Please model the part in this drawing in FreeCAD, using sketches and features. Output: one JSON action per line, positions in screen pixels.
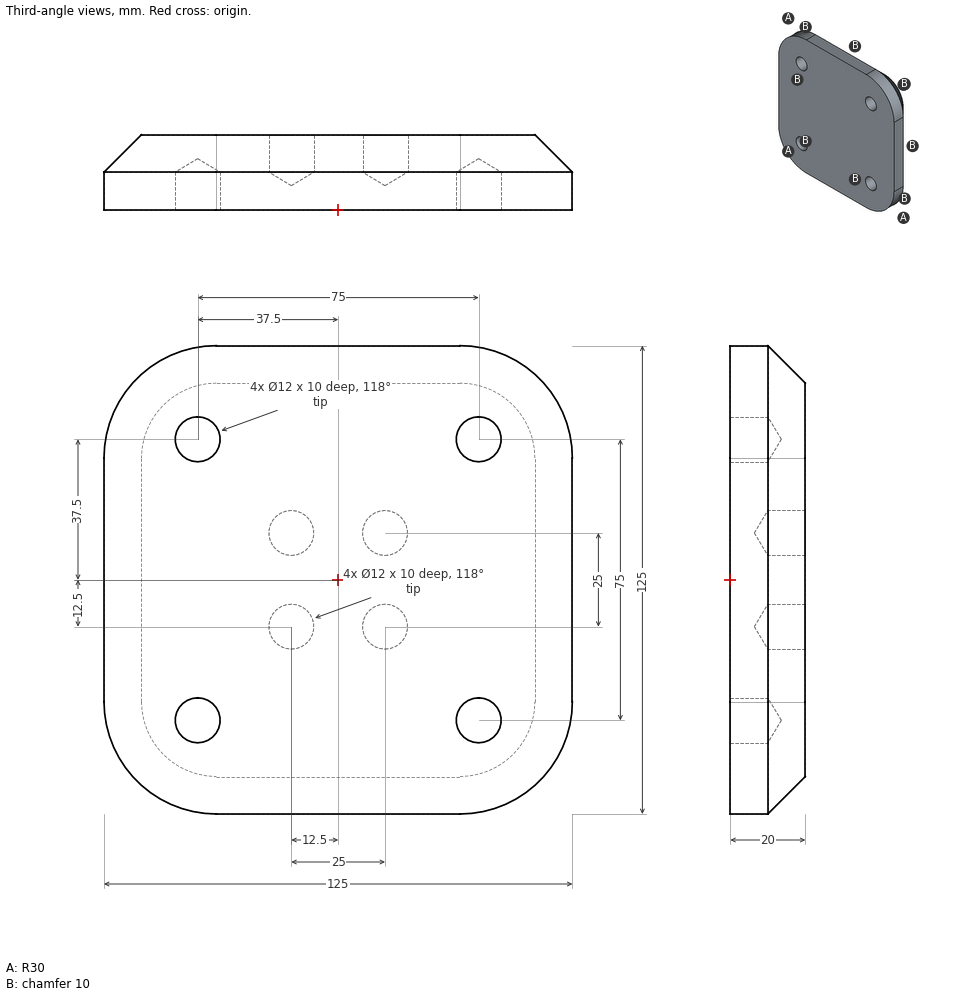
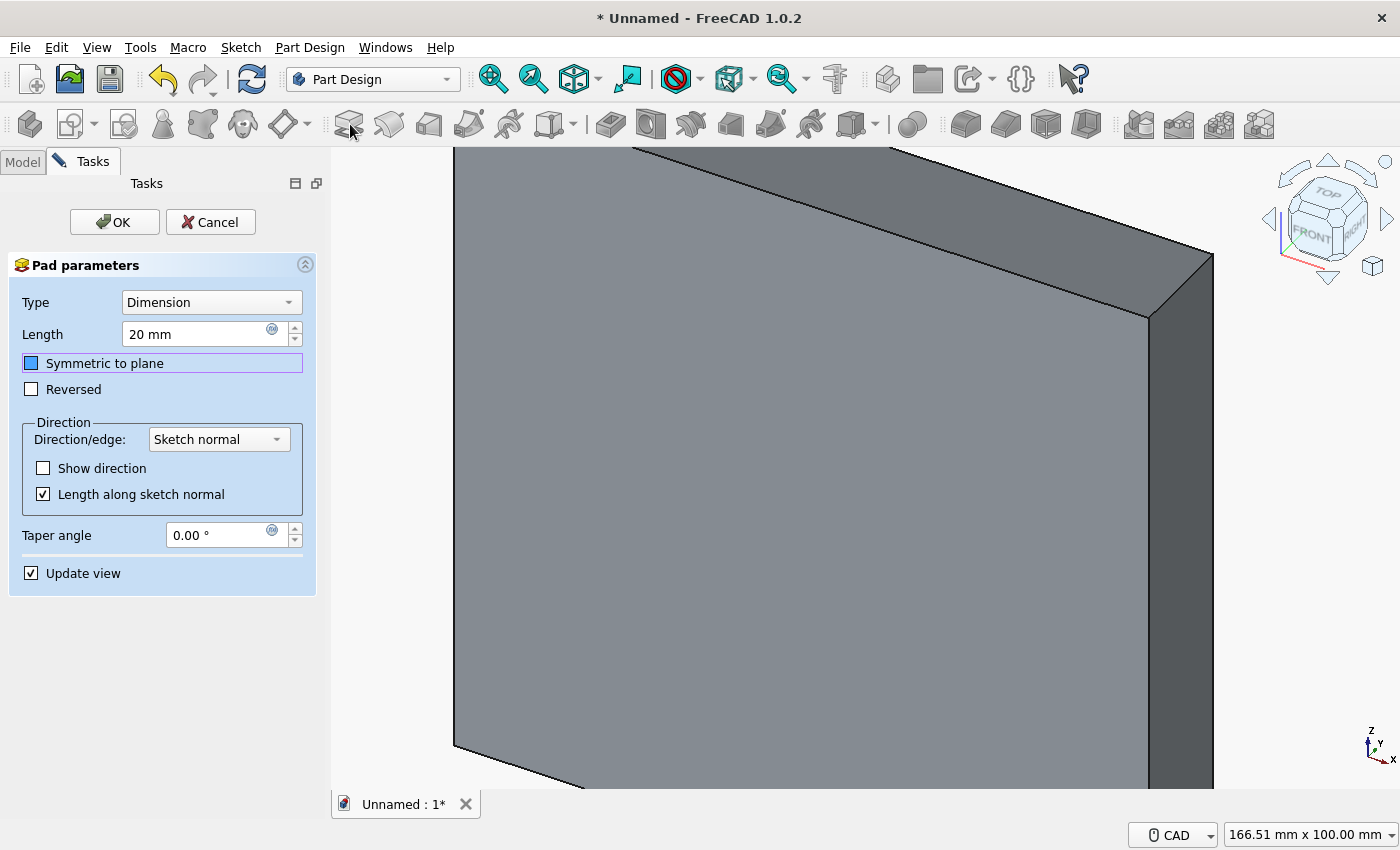
{"action": "left_click", "coordinate": [30, 389]}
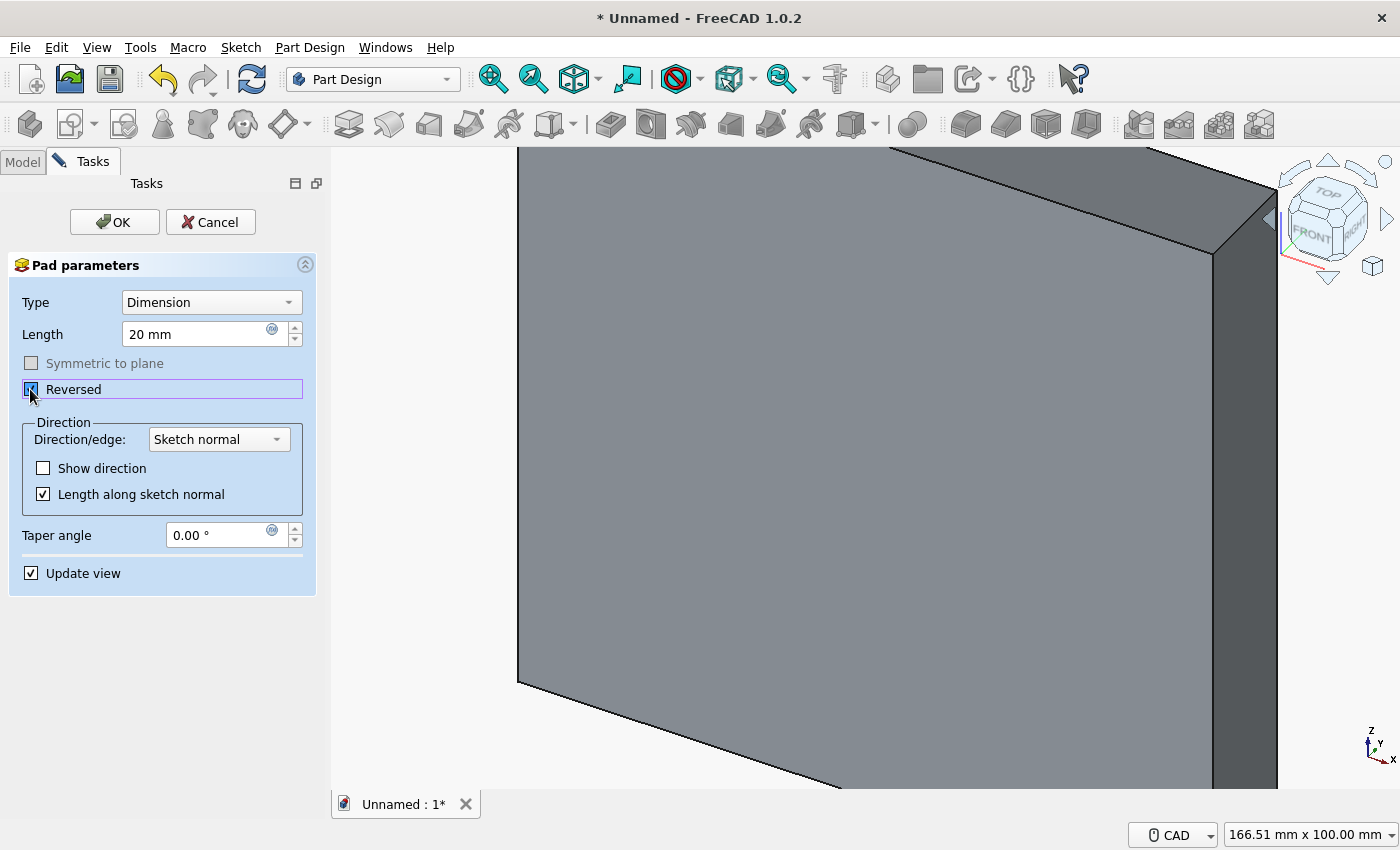
{"action": "left_click", "coordinate": [115, 222]}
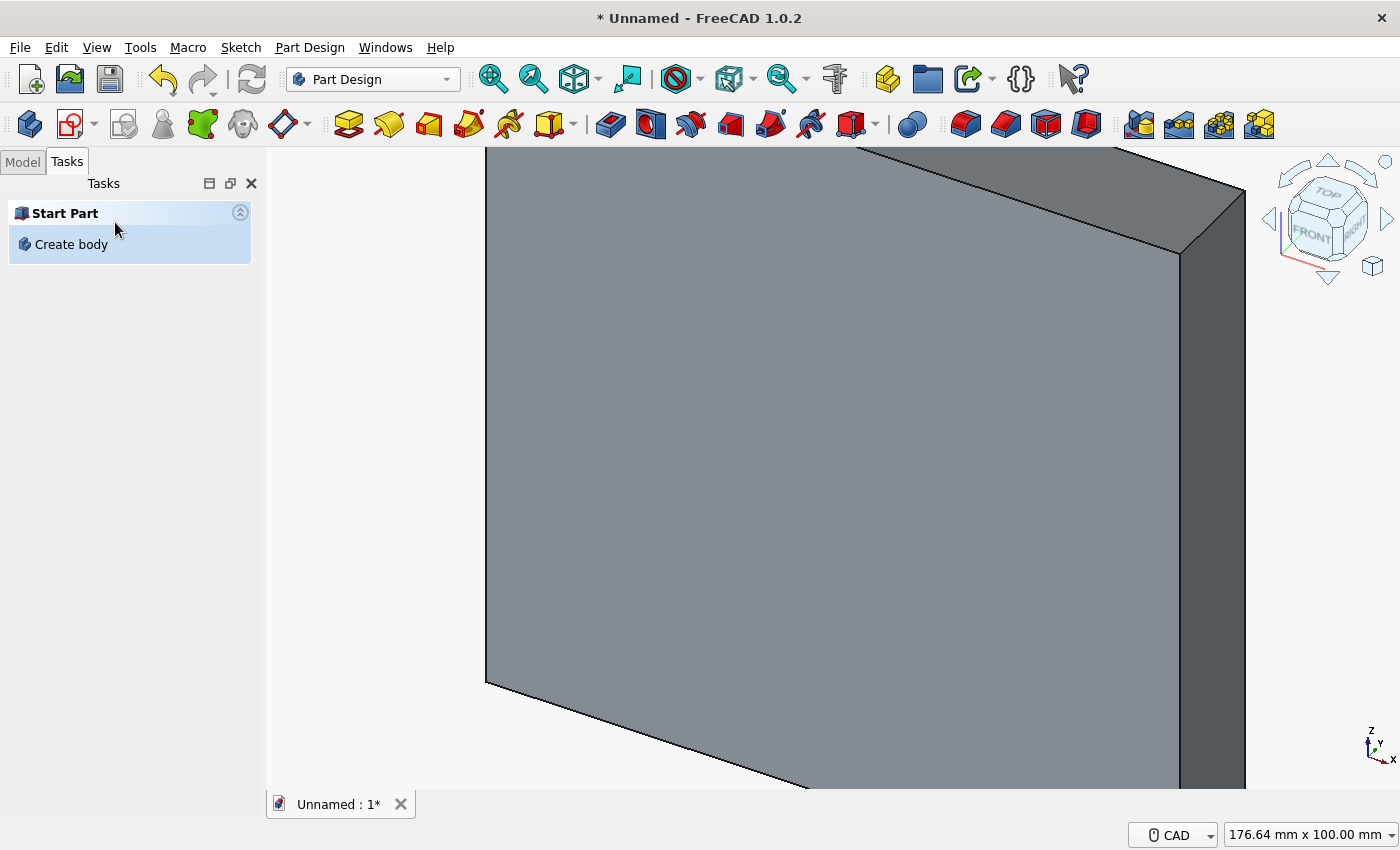
{"action": "key", "text": "v f"}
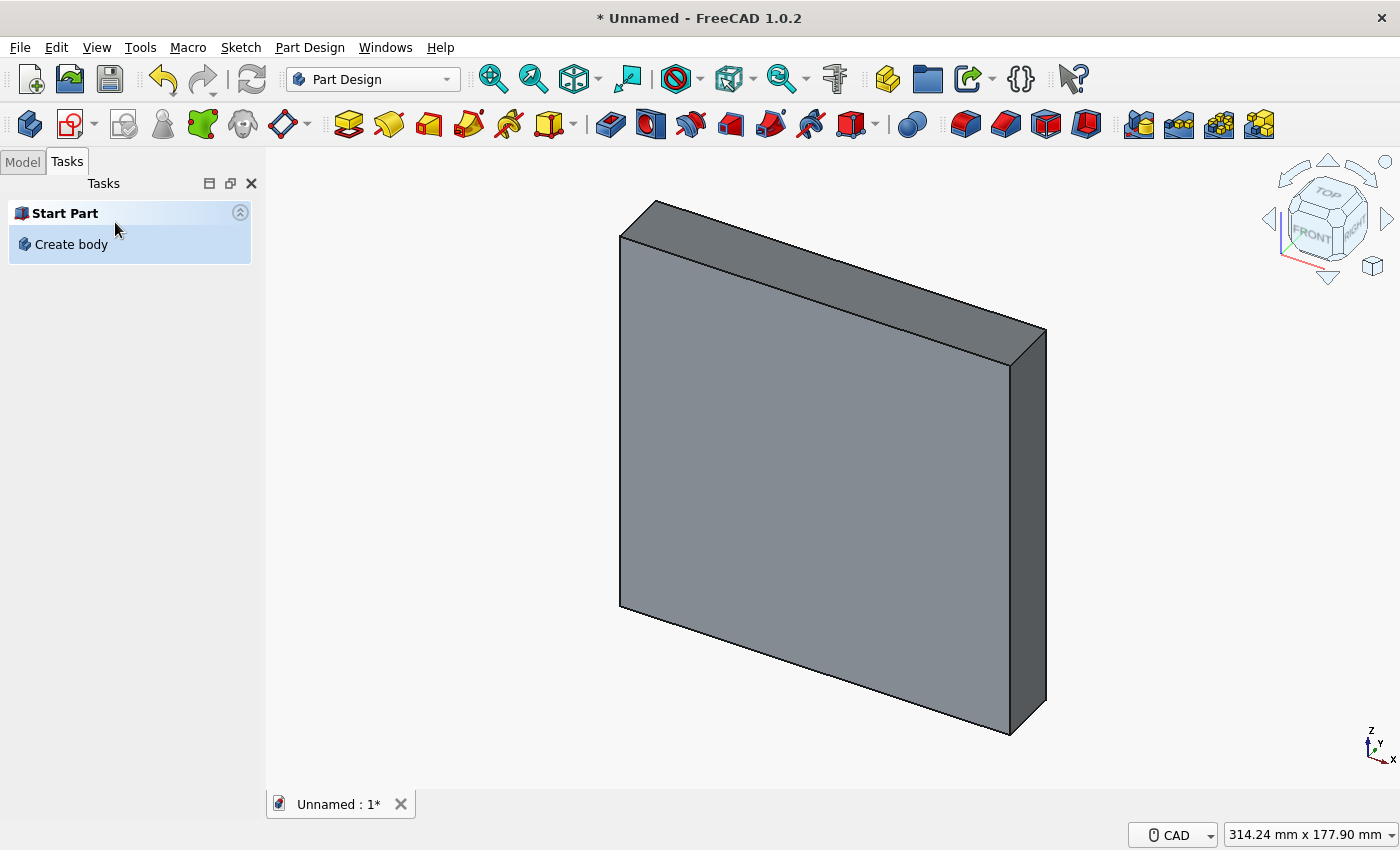
{"action": "left_click", "coordinate": [1028, 347]}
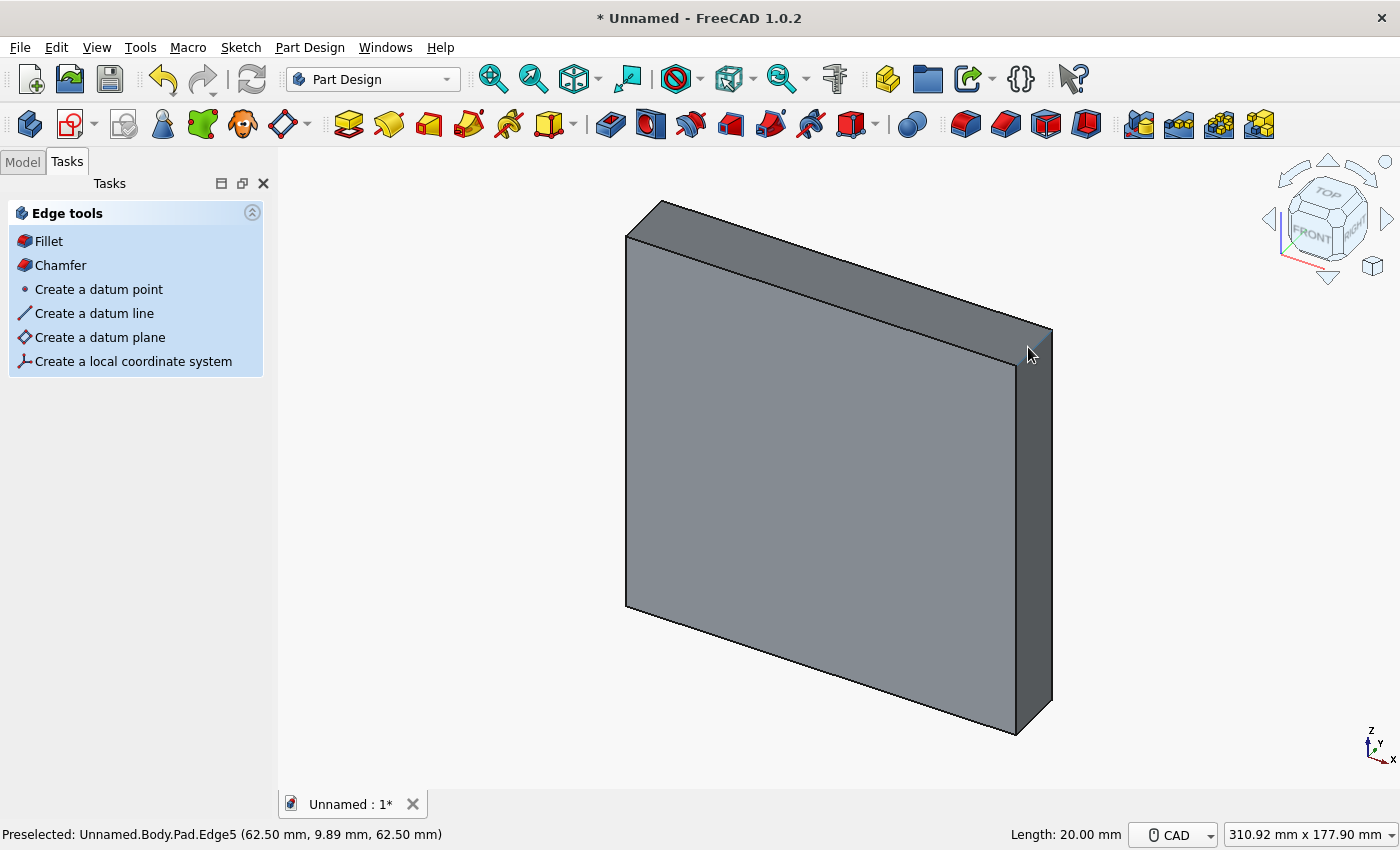
{"action": "key", "text": "0"}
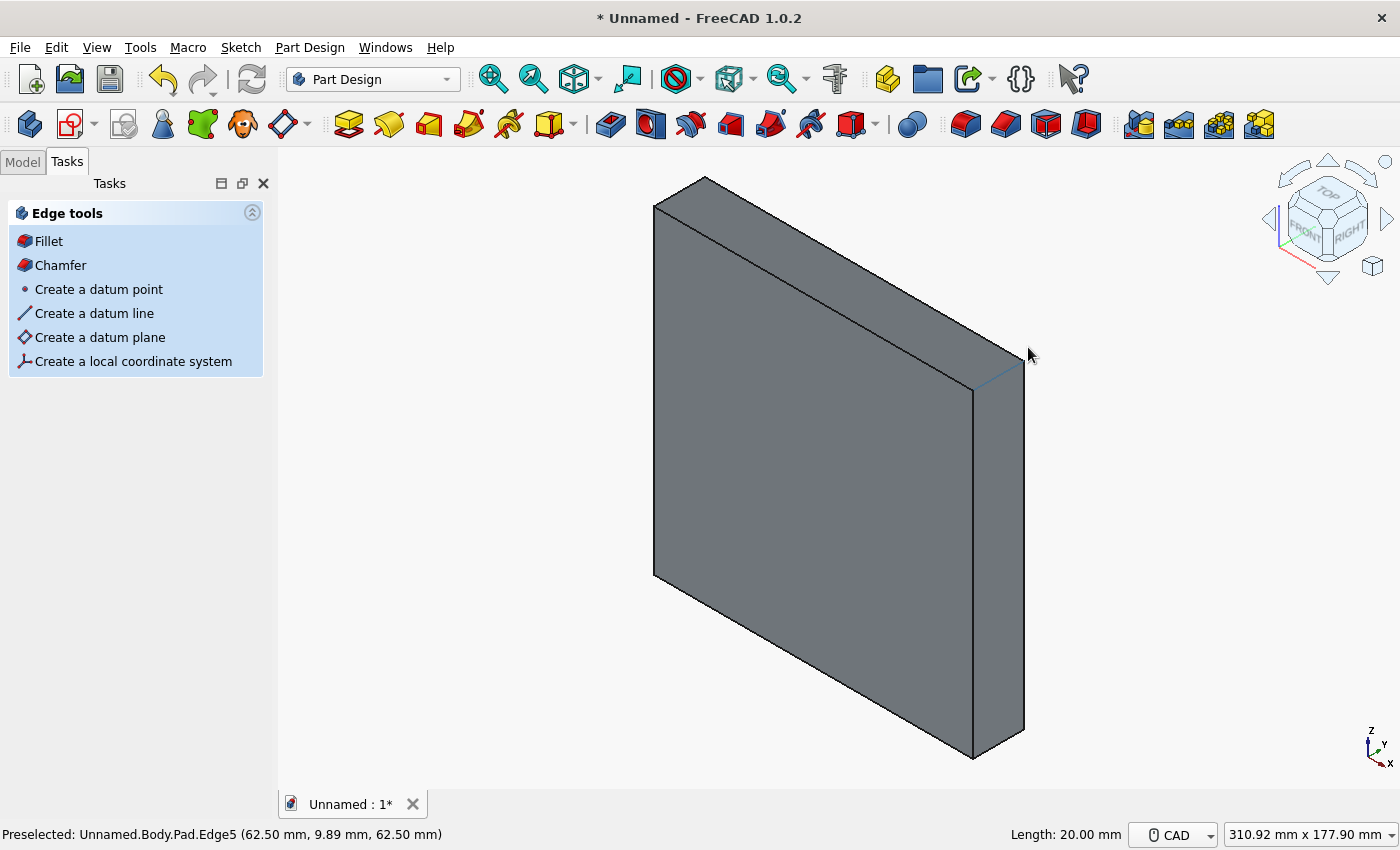
{"action": "key", "text": "2"}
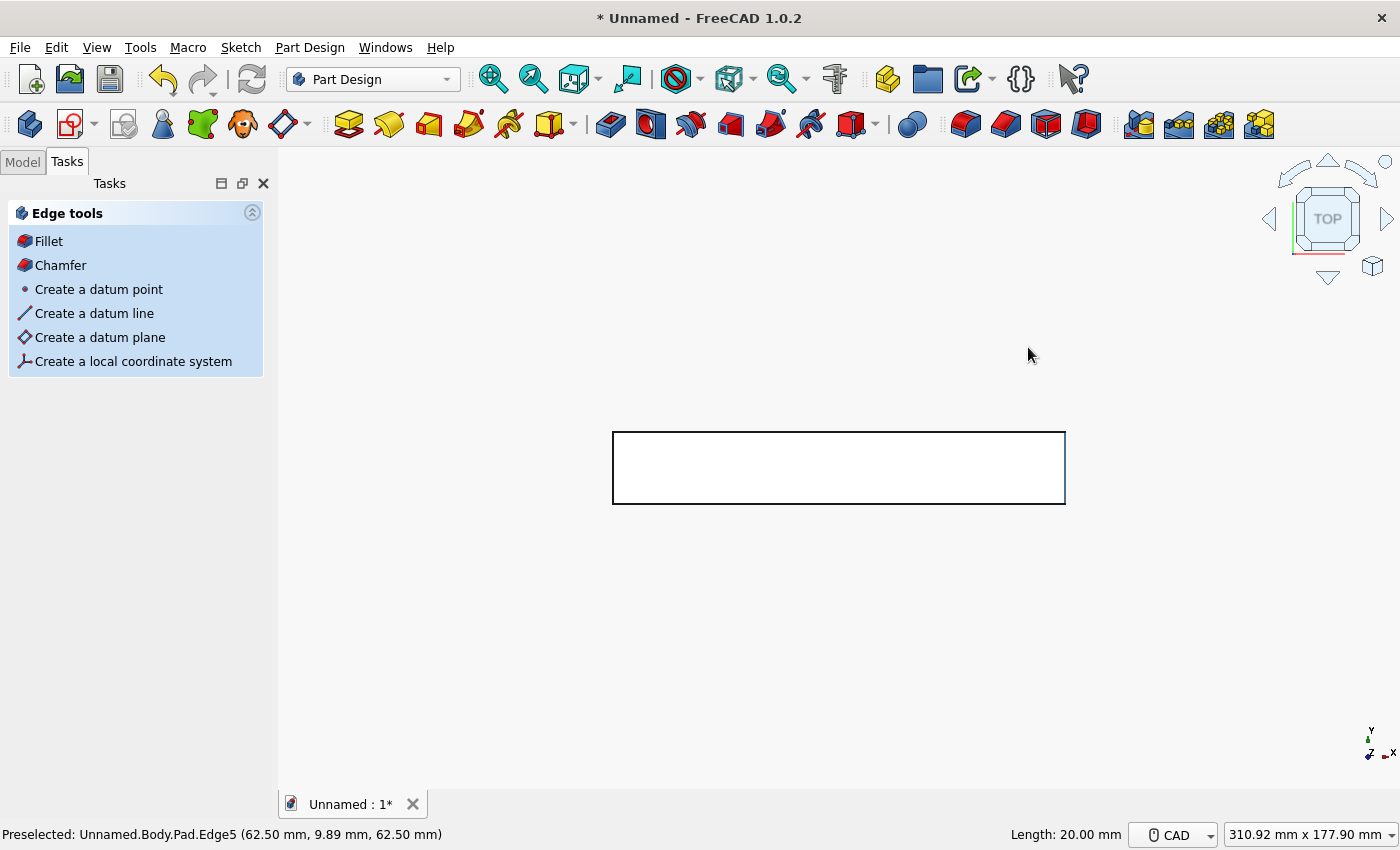
{"action": "key", "text": "v f"}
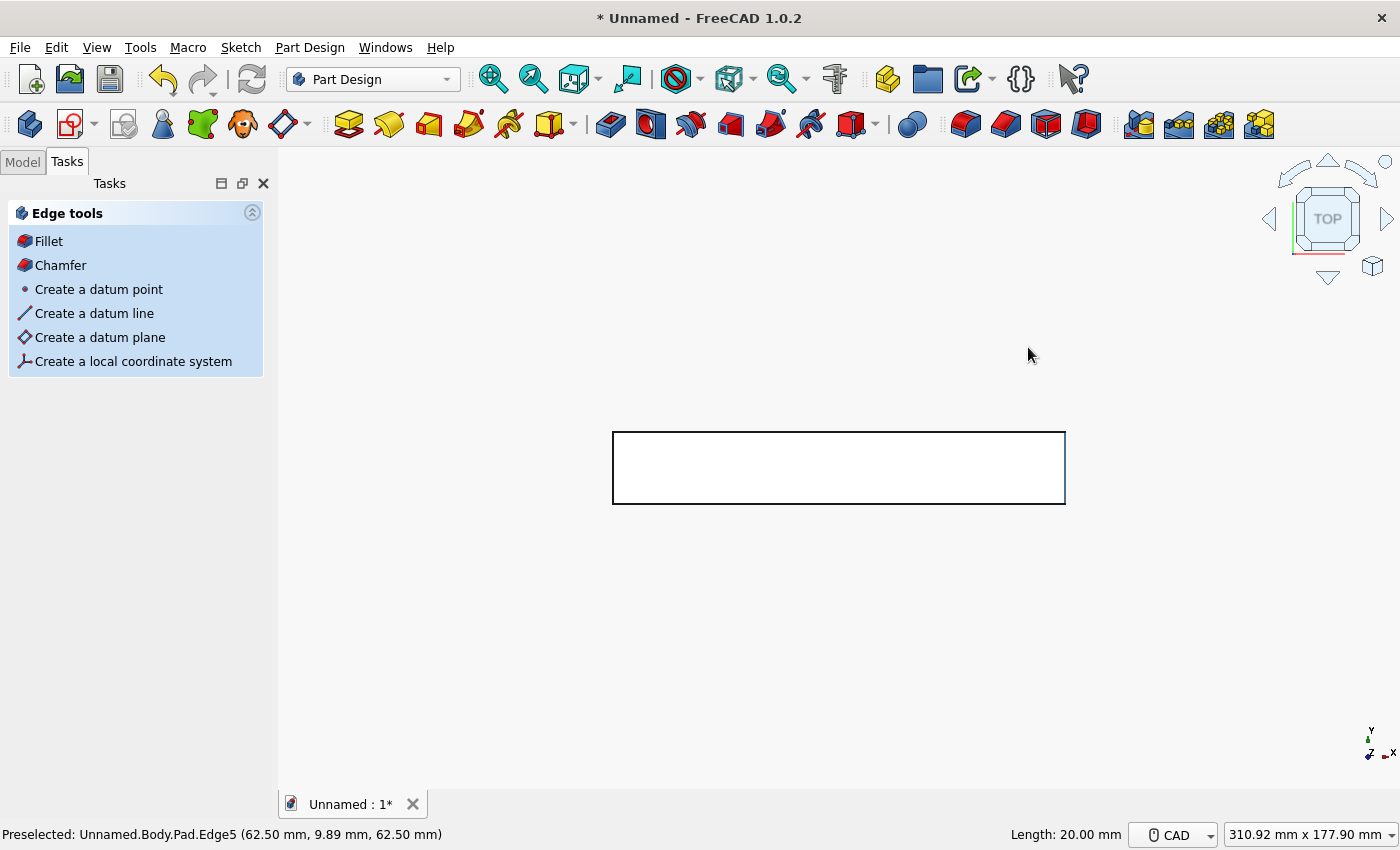
{"action": "left_click", "coordinate": [613, 467], "text": "ctrl"}